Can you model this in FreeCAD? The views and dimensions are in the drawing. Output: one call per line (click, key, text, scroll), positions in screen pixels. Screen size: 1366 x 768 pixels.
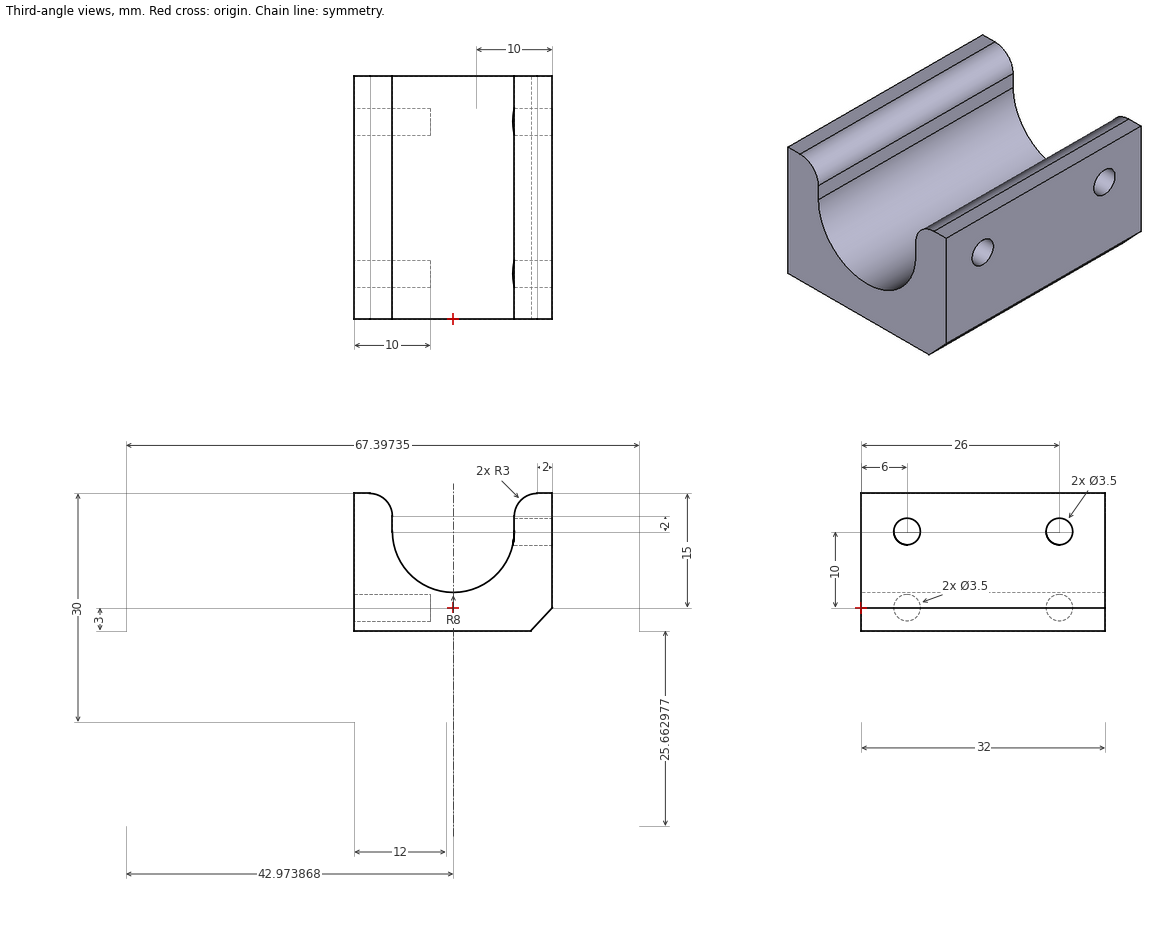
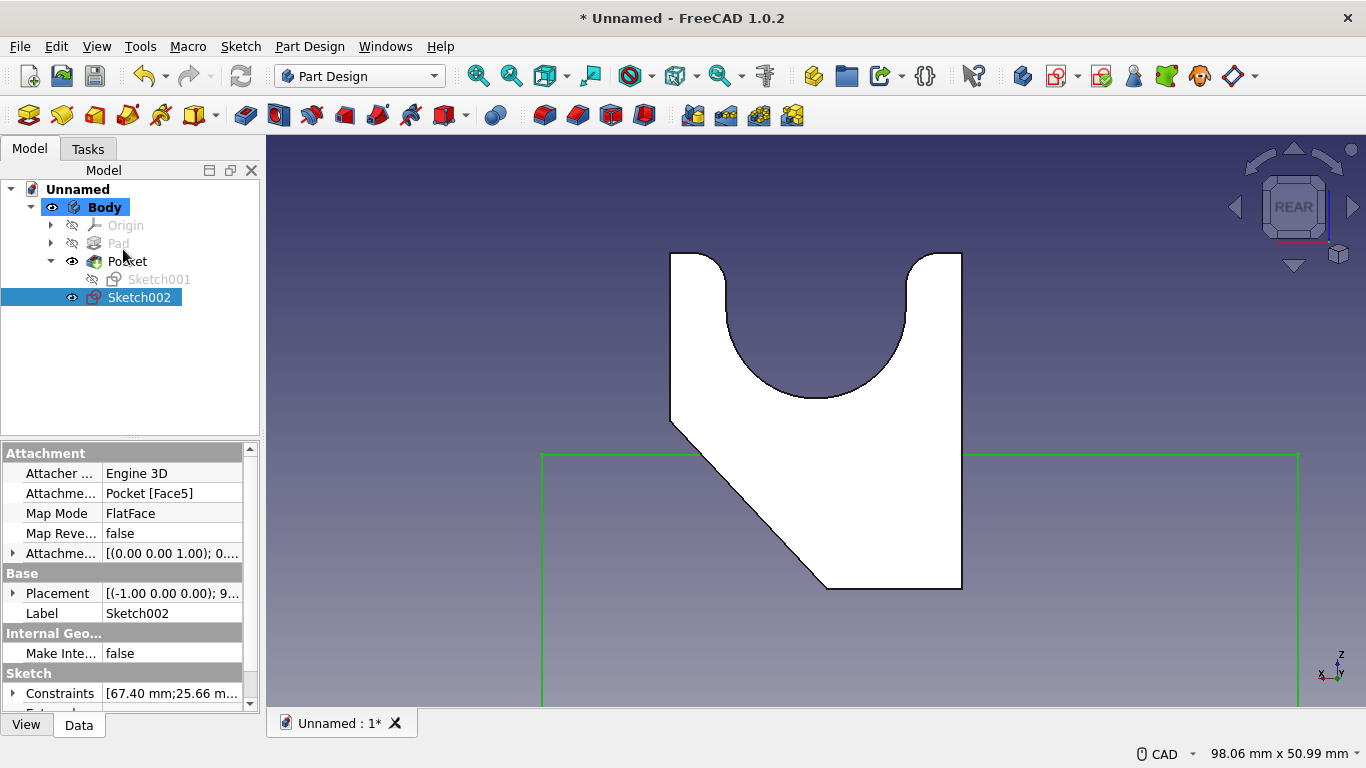
click(246, 116)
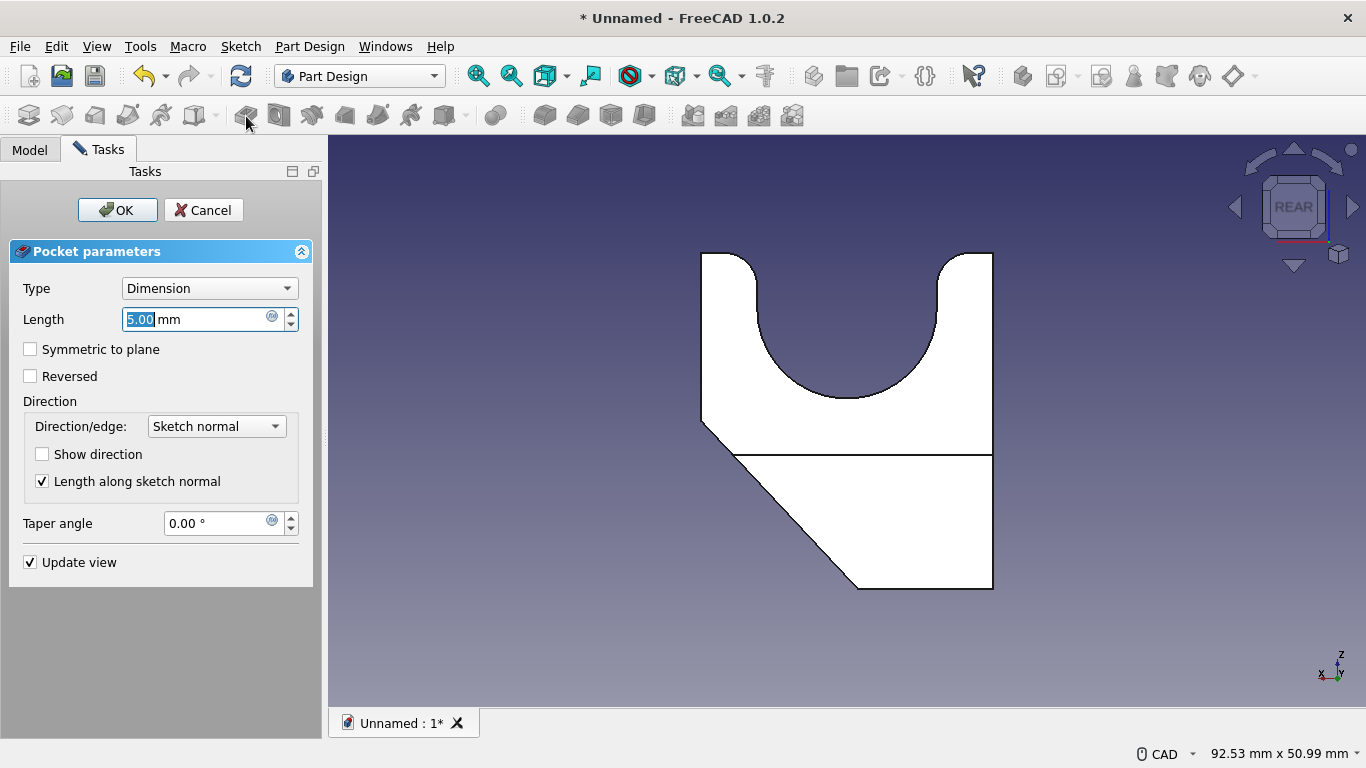
click(210, 288)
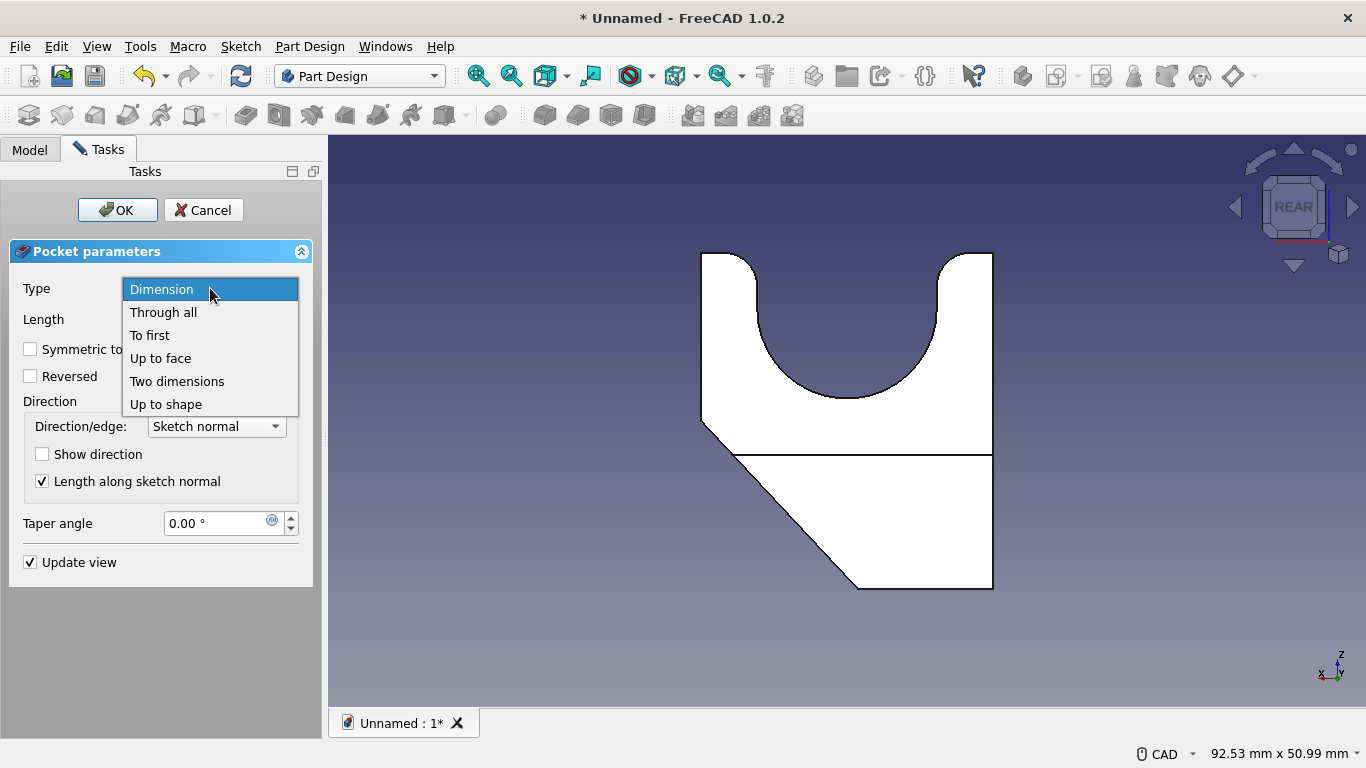
click(208, 312)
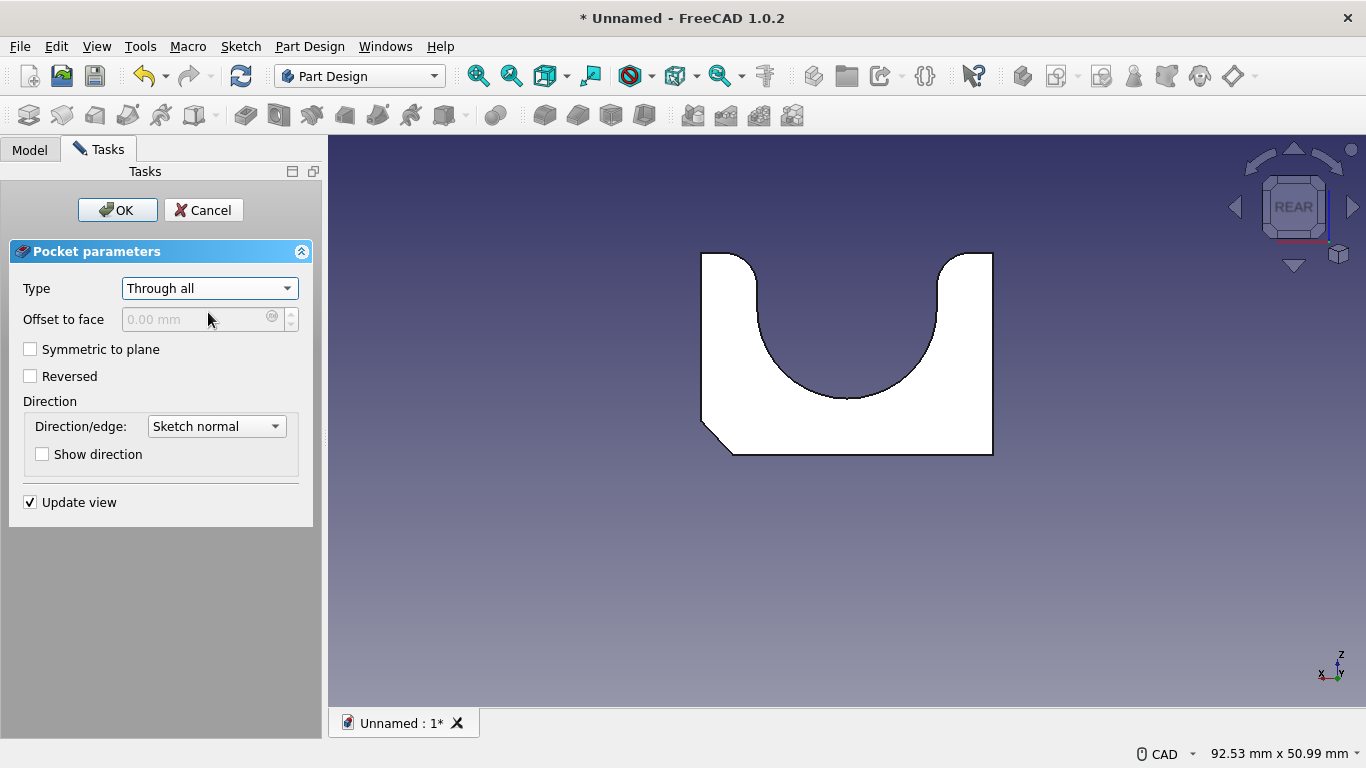
click(118, 210)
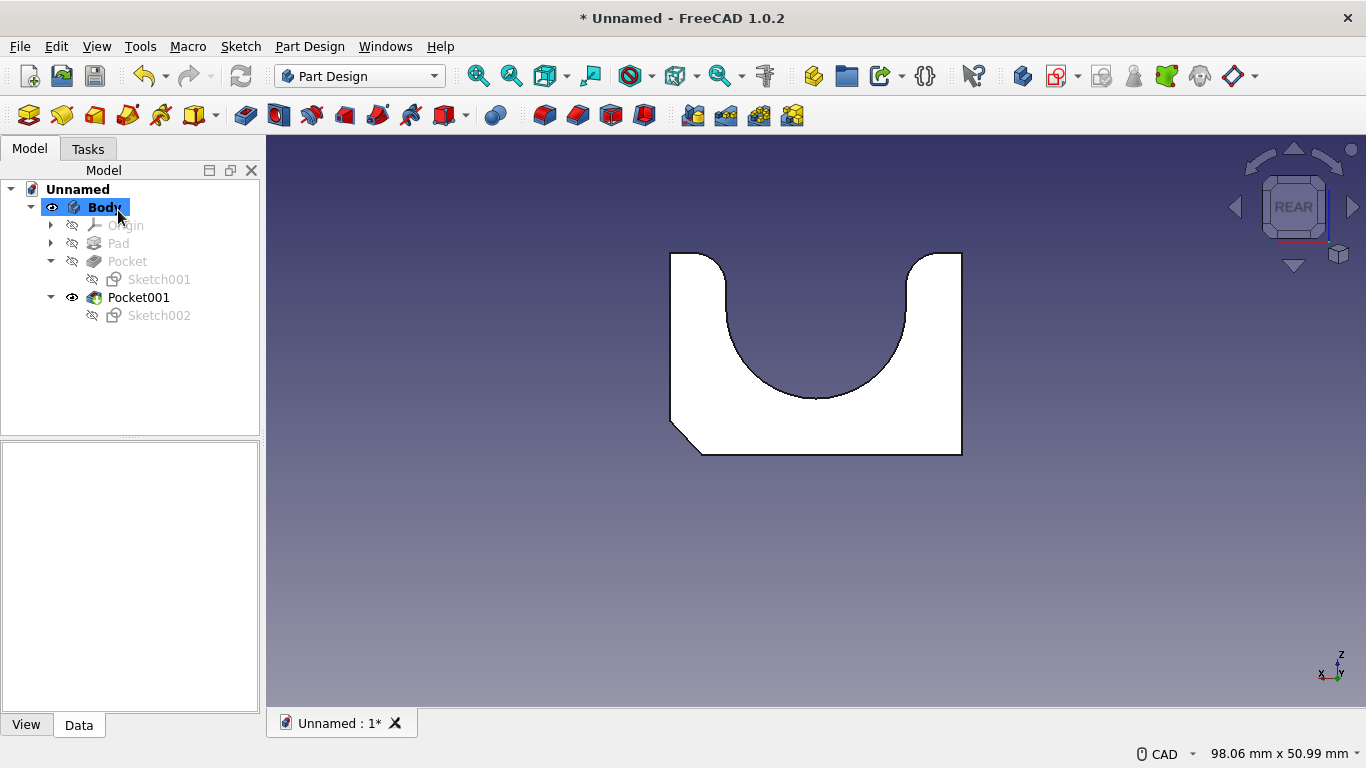
click(479, 76)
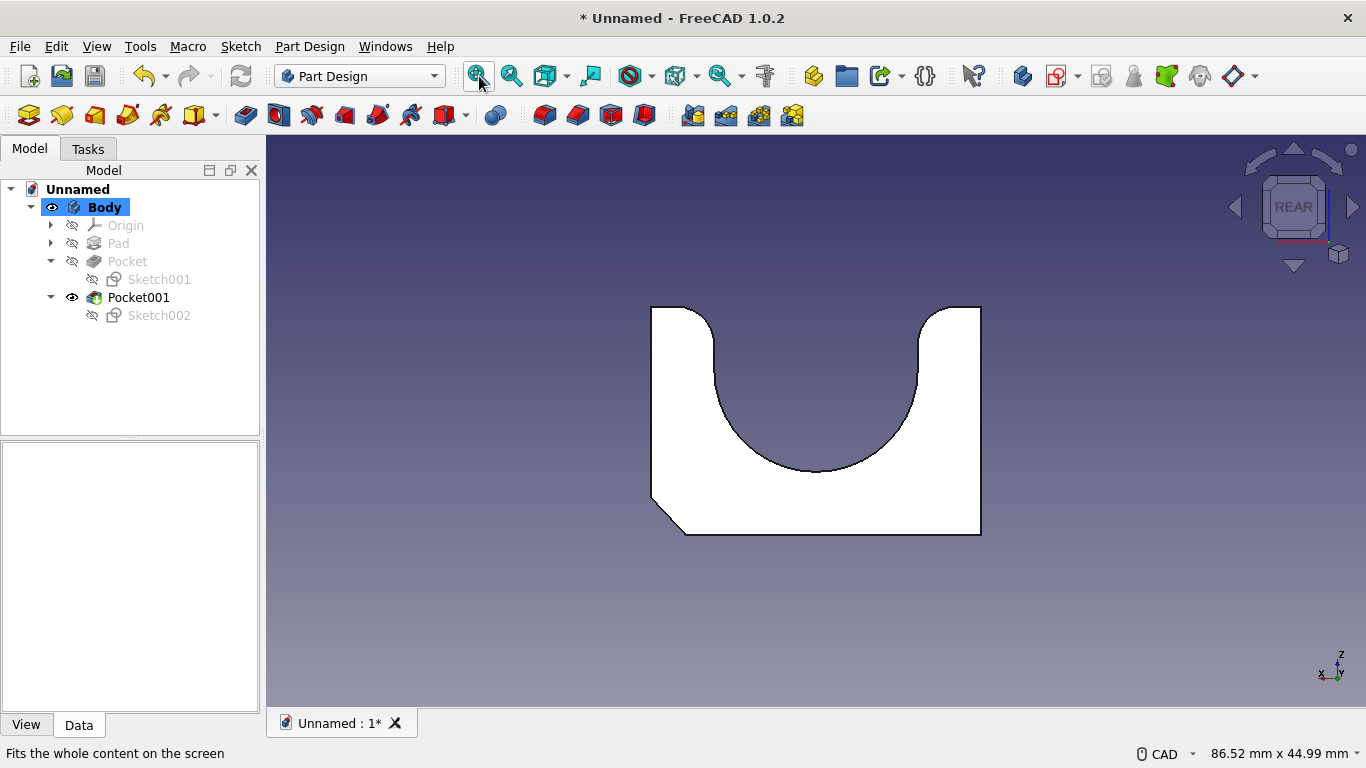
key(6)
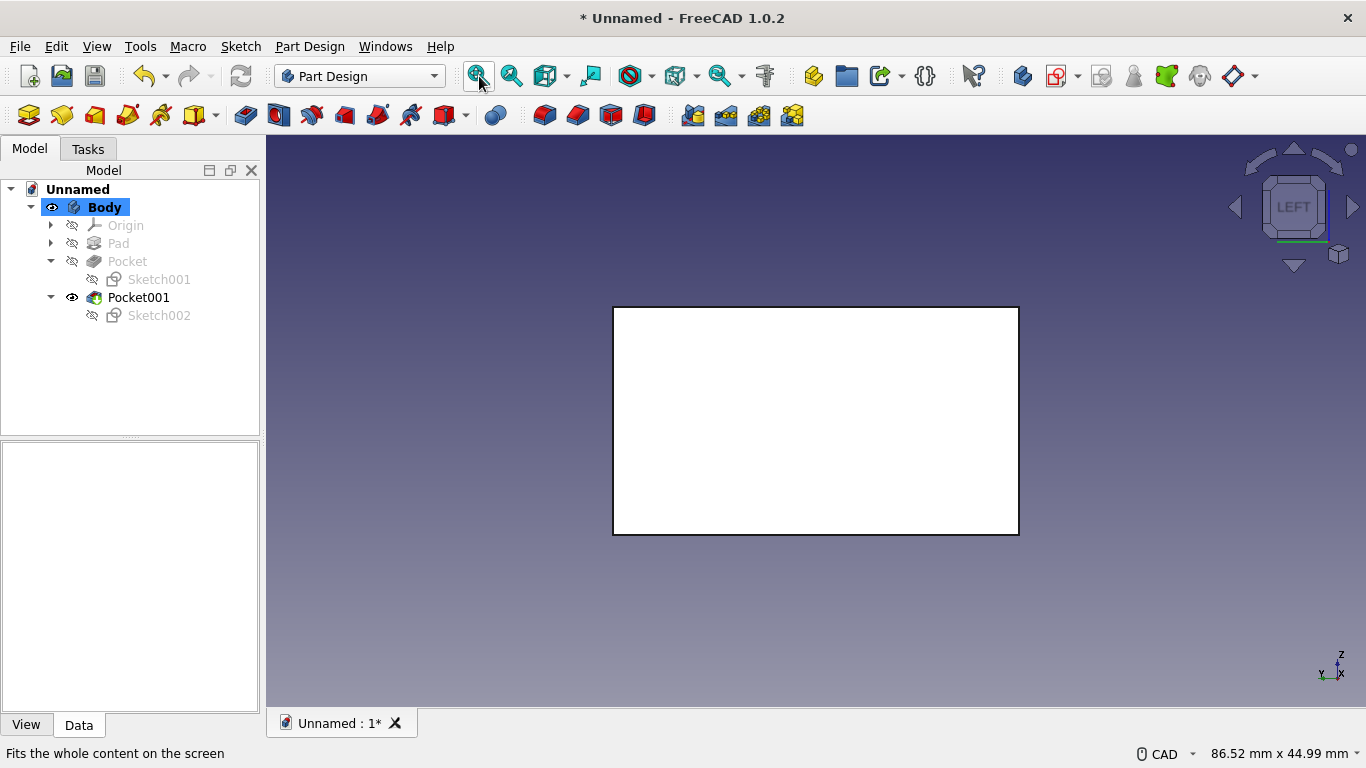
click(479, 76)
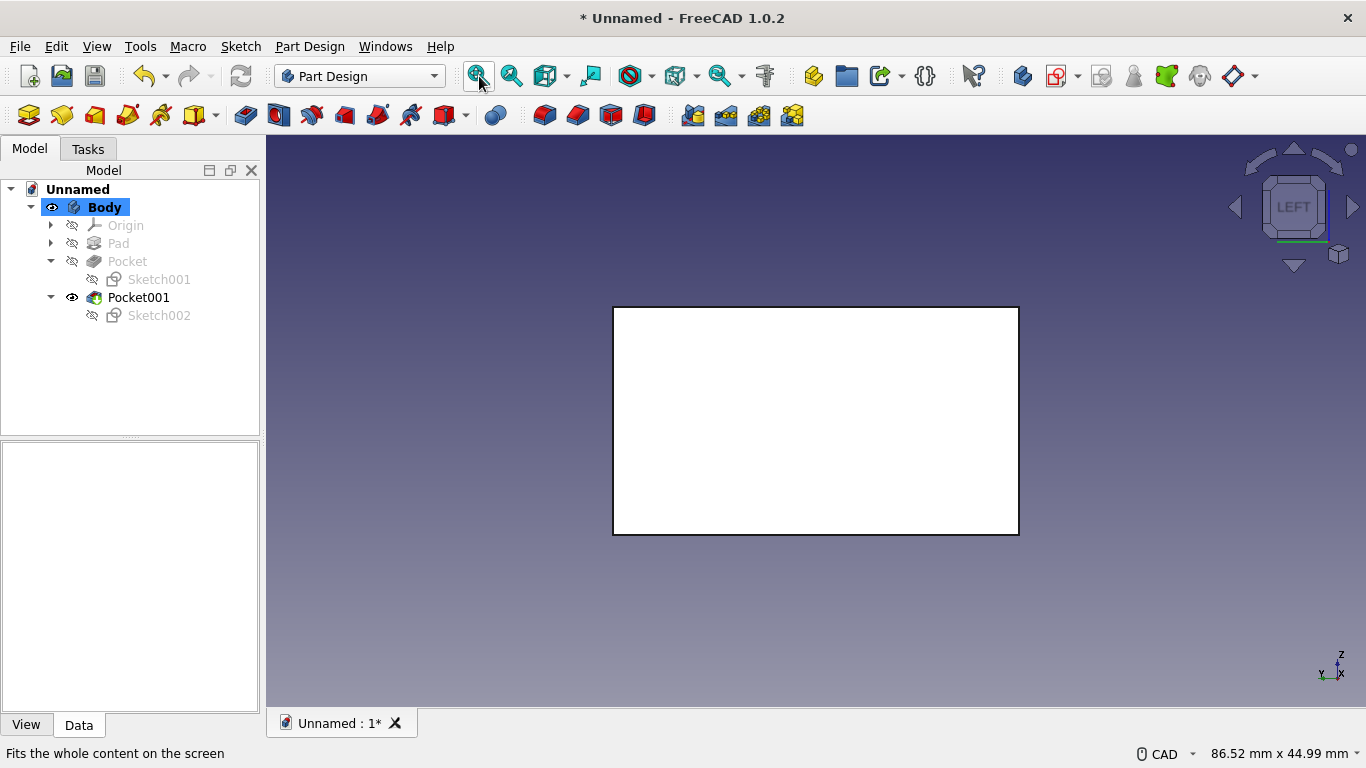
click(874, 420)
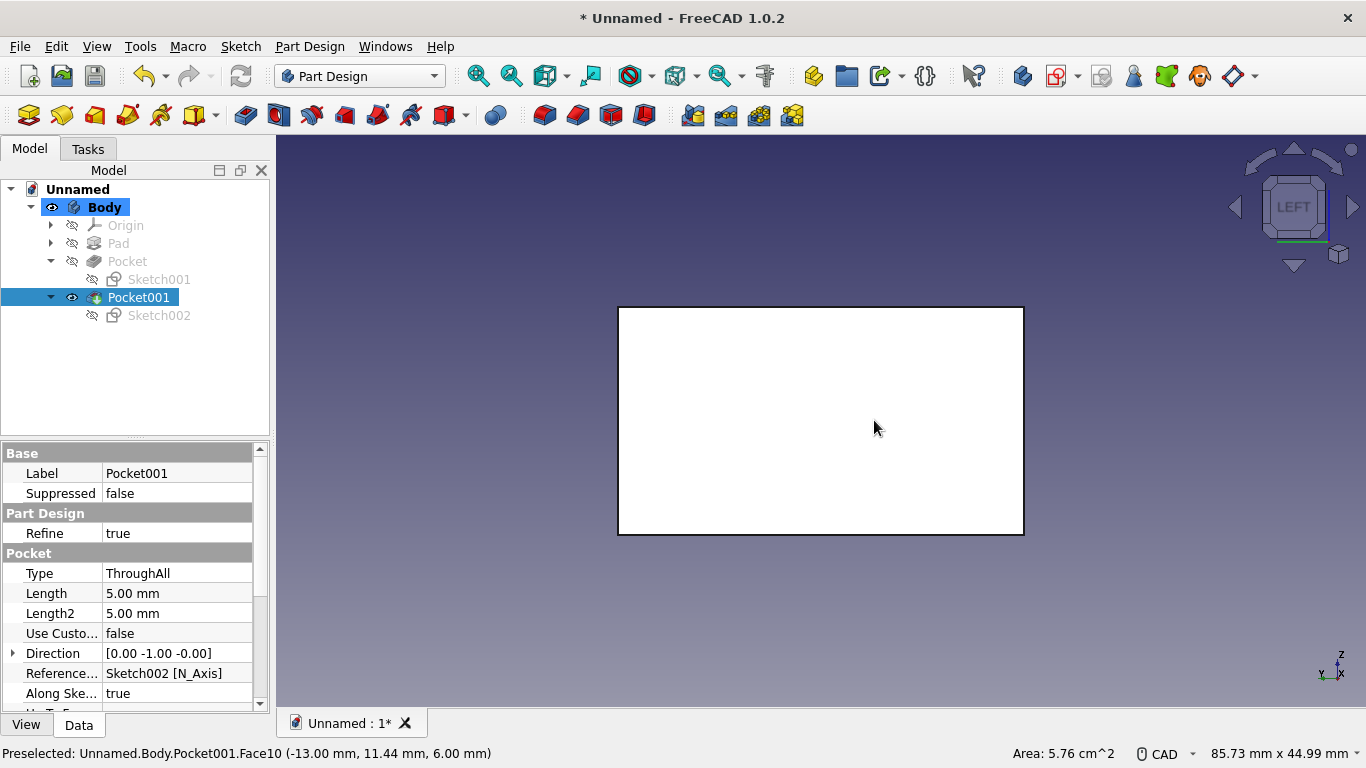
click(1056, 76)